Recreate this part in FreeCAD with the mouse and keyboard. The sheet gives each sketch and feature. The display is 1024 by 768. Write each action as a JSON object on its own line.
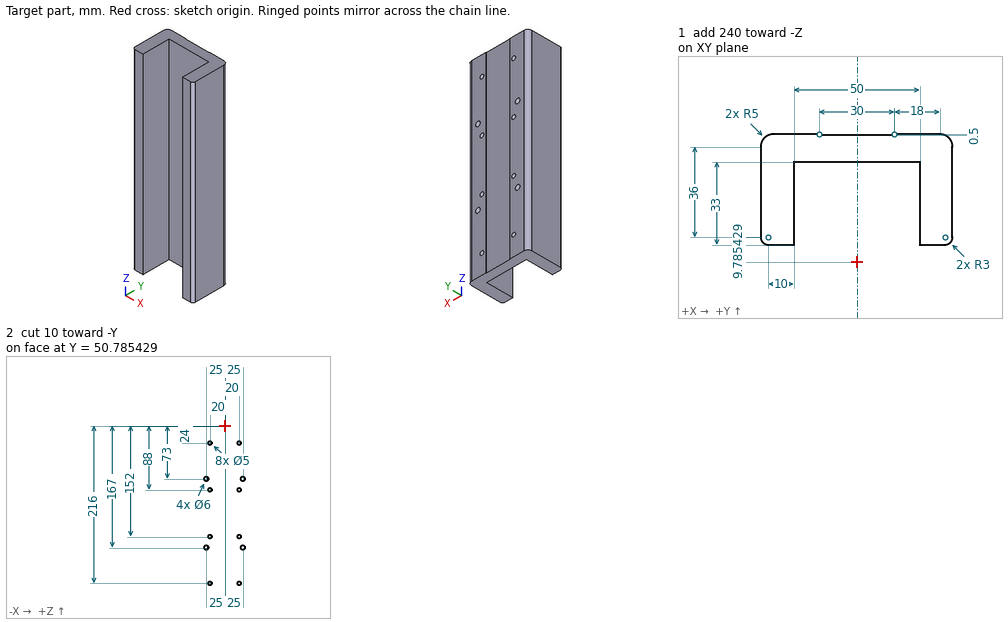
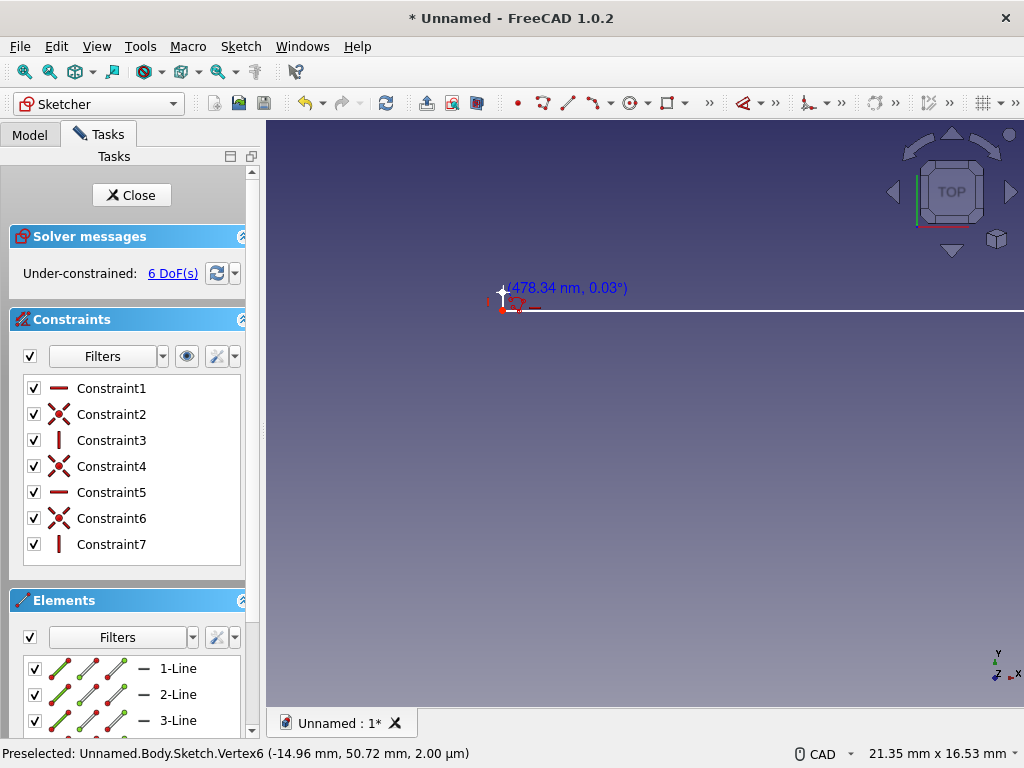
{"action": "scroll", "coordinate": [505, 291], "scroll_direction": "down", "scroll_amount": 10}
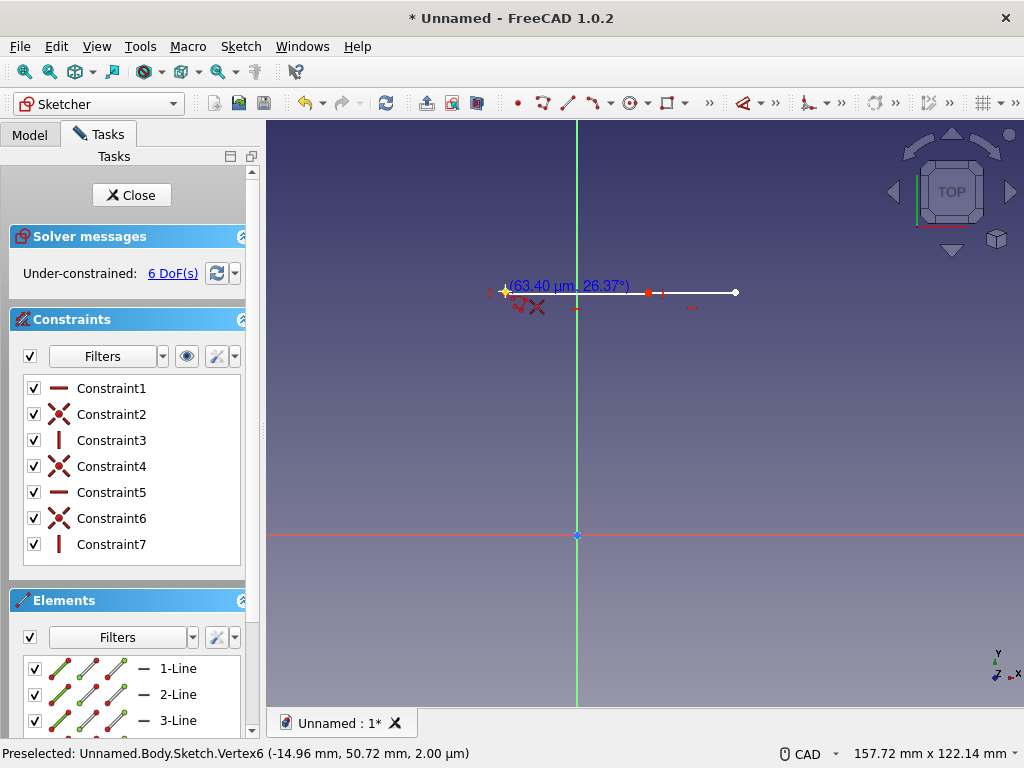
{"action": "left_click", "coordinate": [418, 291]}
{"action": "right_click", "coordinate": [418, 291]}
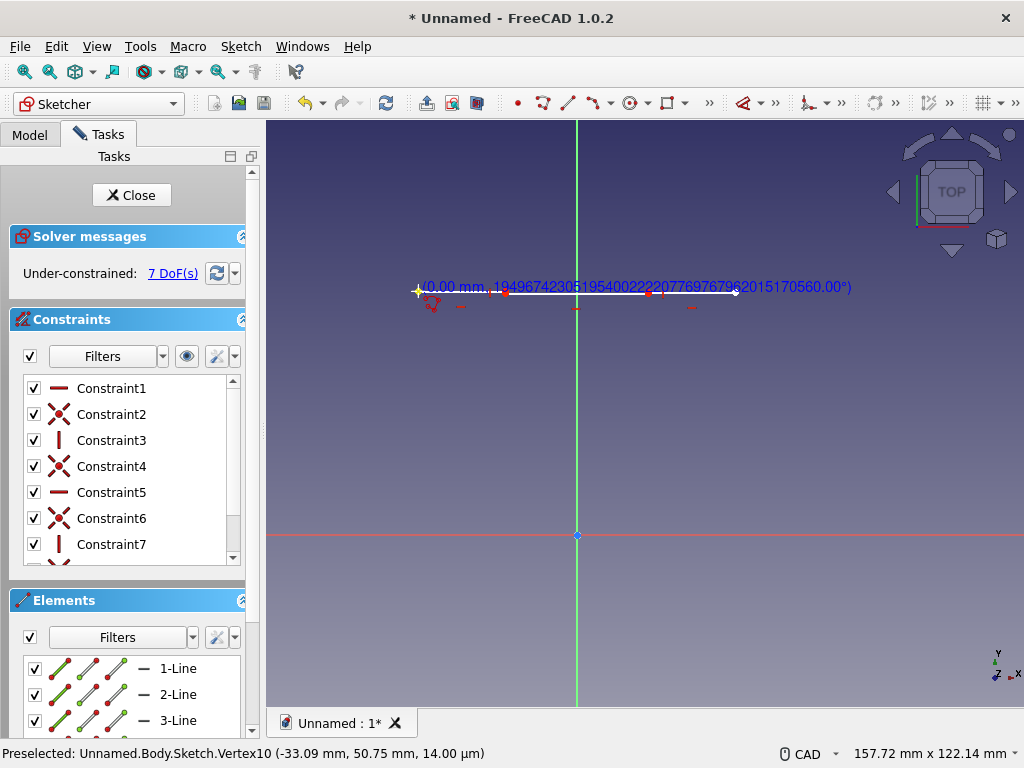
{"action": "left_click", "coordinate": [568, 104]}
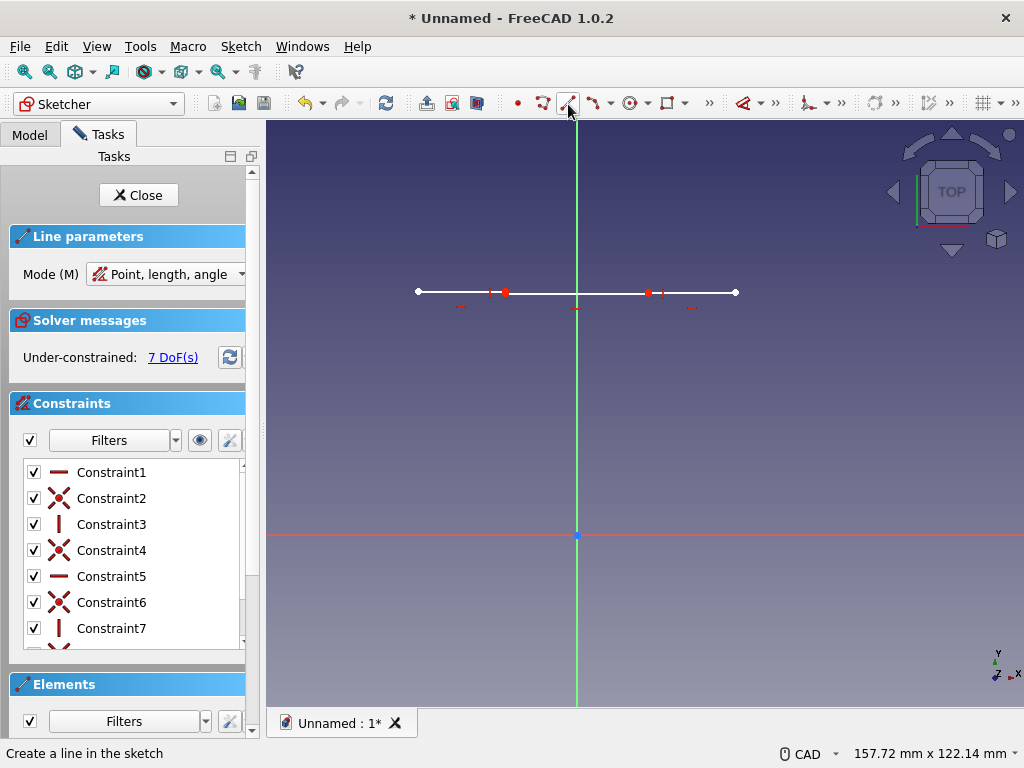
{"action": "left_click", "coordinate": [394, 315]}
{"action": "left_click", "coordinate": [394, 488]}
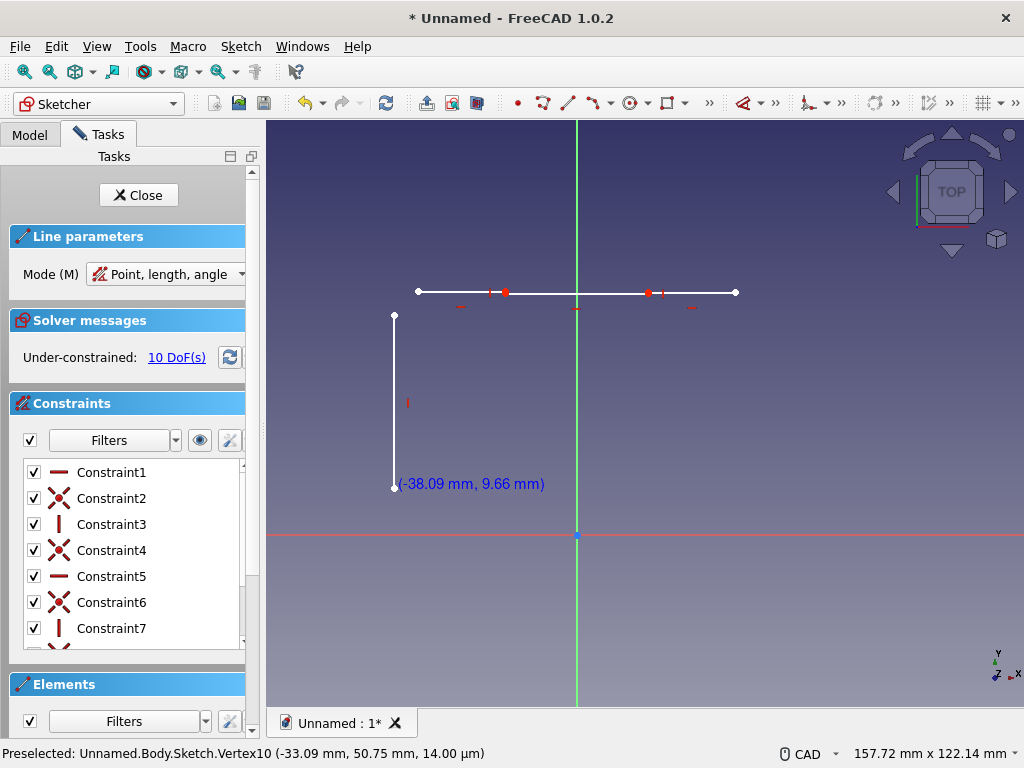
{"action": "left_click", "coordinate": [543, 104]}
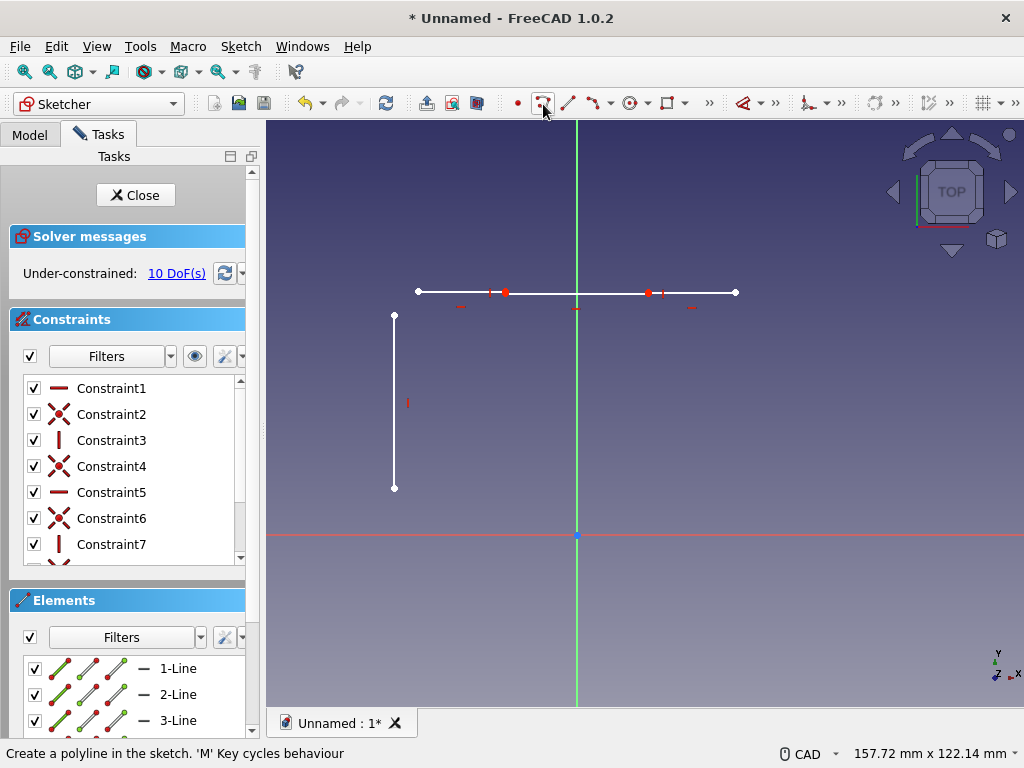
{"action": "left_click", "coordinate": [409, 503]}
{"action": "left_click", "coordinate": [457, 503]}
{"action": "left_click", "coordinate": [457, 344]}
{"action": "left_click", "coordinate": [697, 344]}
{"action": "left_click", "coordinate": [697, 503]}
{"action": "left_click", "coordinate": [745, 503]}
{"action": "right_click", "coordinate": [745, 503]}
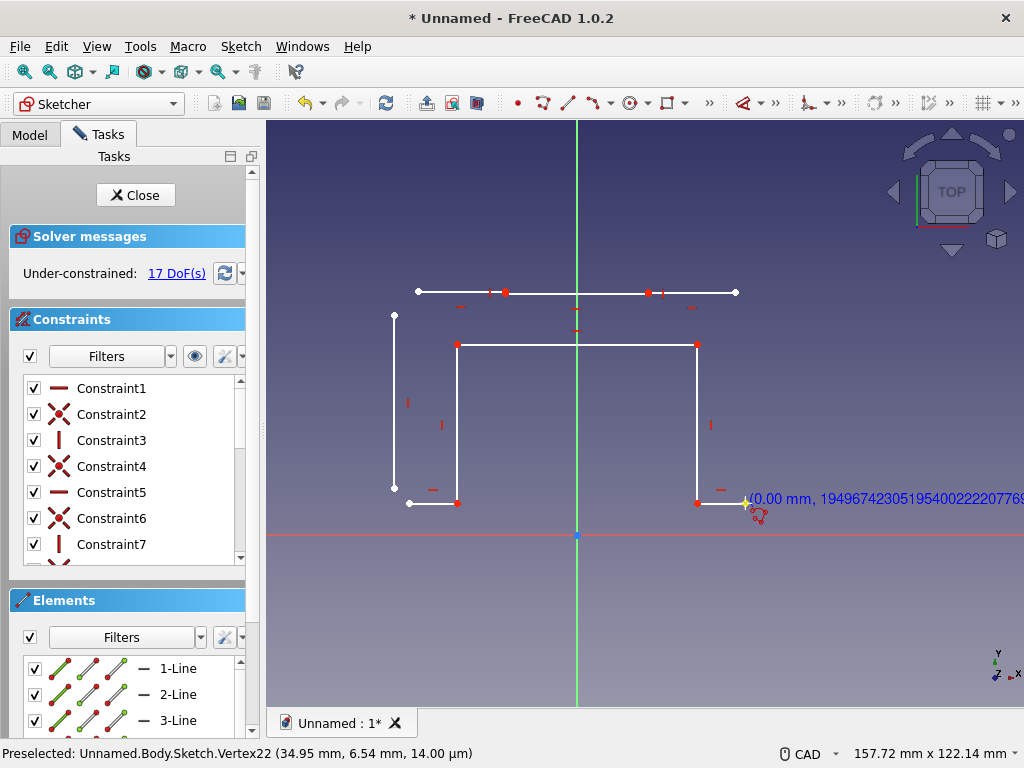
{"action": "left_click", "coordinate": [568, 104]}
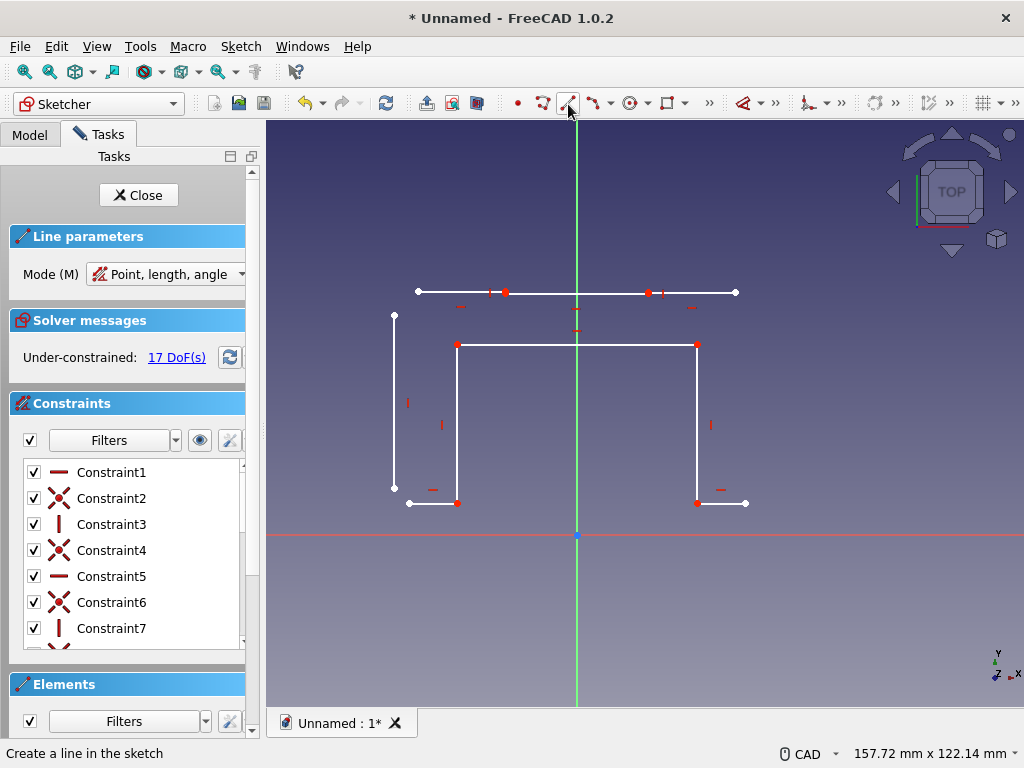
{"action": "left_click", "coordinate": [760, 488]}
{"action": "left_click", "coordinate": [760, 315]}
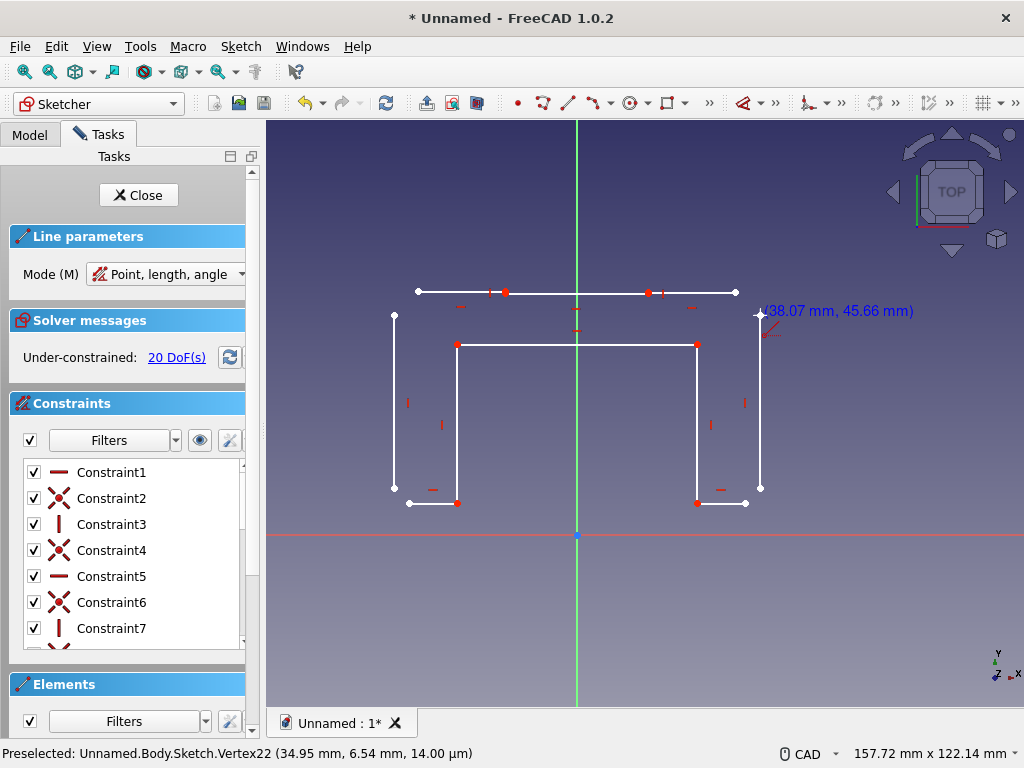
{"action": "left_click", "coordinate": [592, 104]}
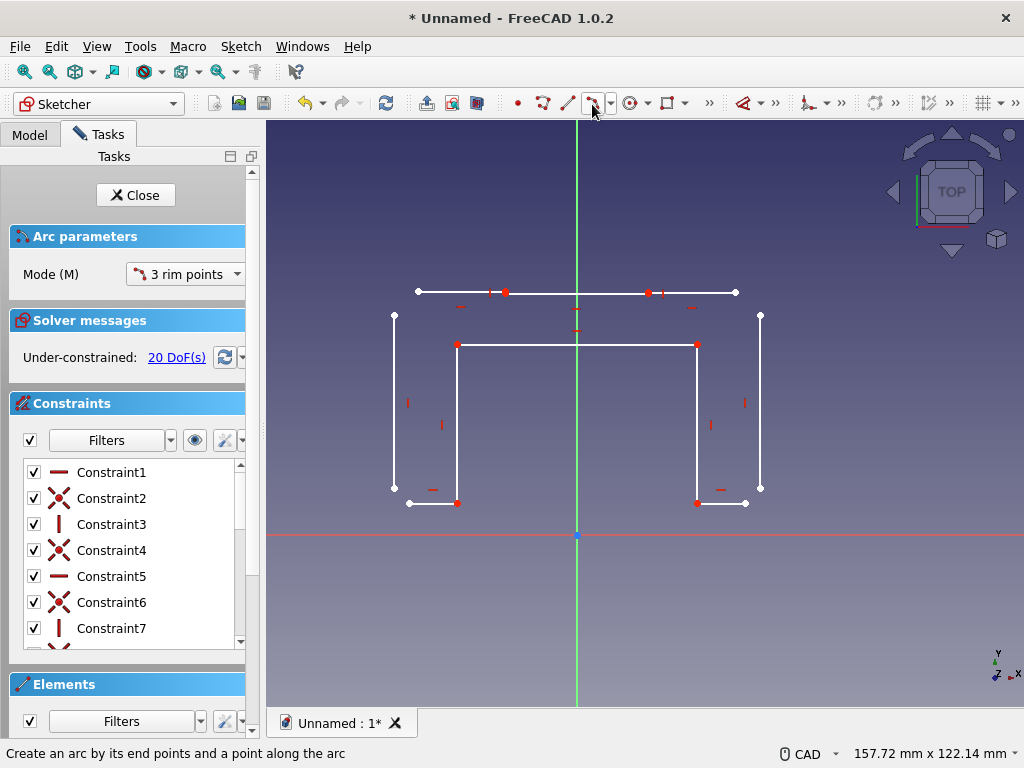
{"action": "left_click", "coordinate": [418, 292]}
{"action": "left_click", "coordinate": [394, 316]}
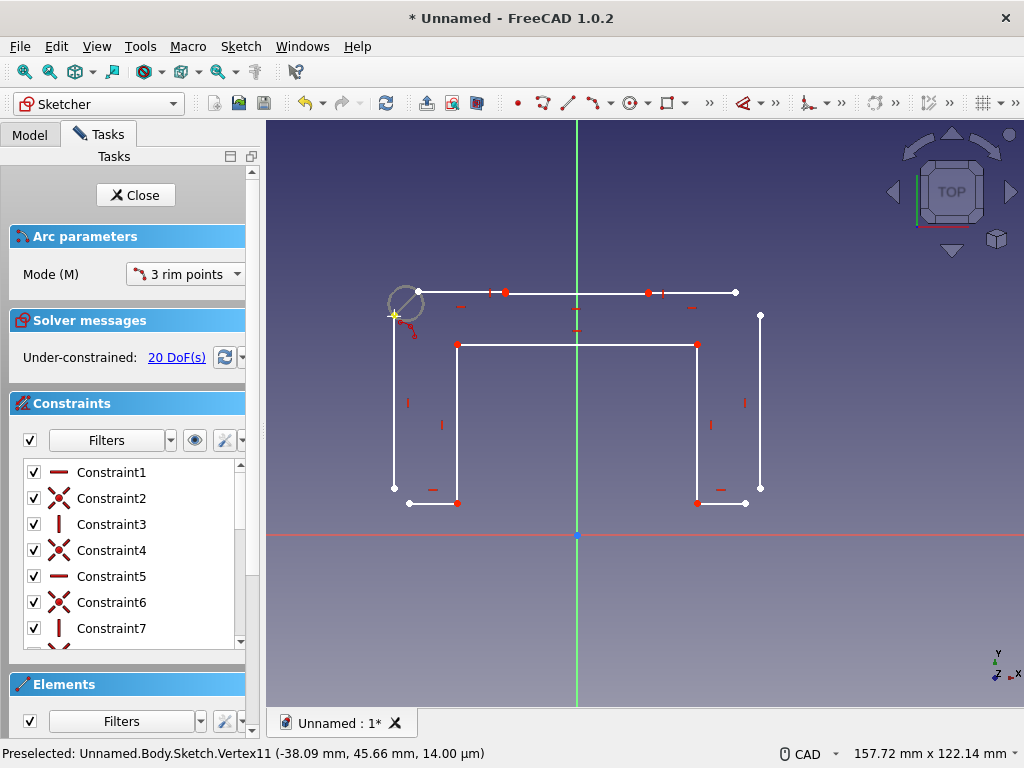
{"action": "scroll", "coordinate": [401, 298], "scroll_direction": "up", "scroll_amount": 5}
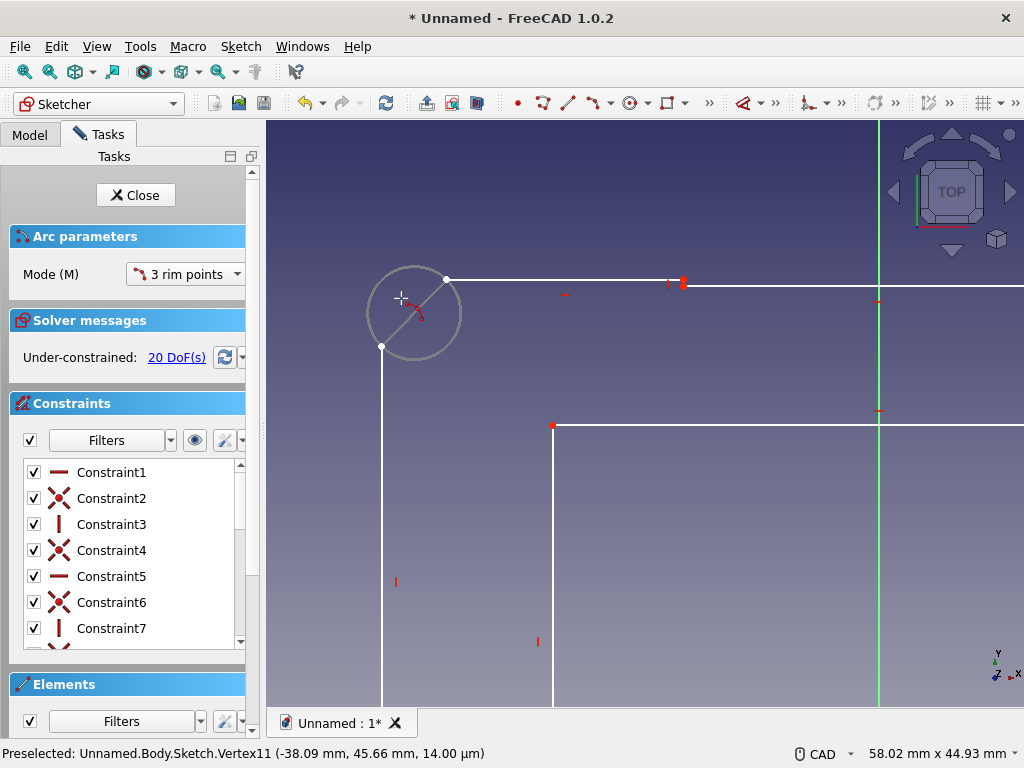
{"action": "left_click", "coordinate": [402, 299]}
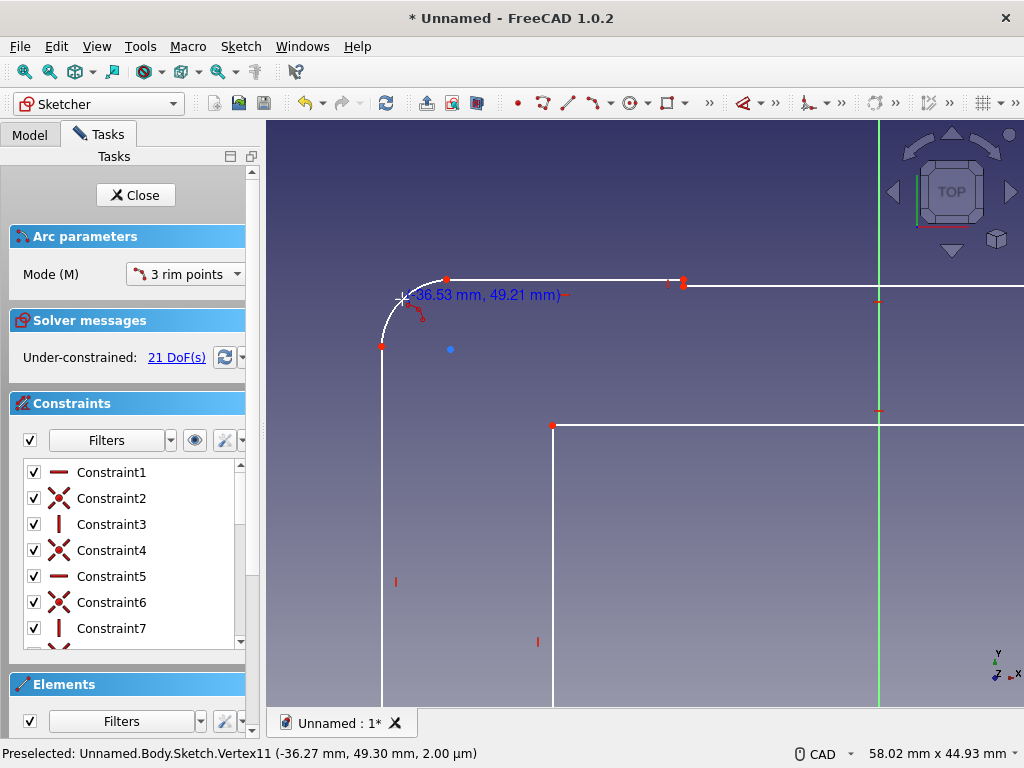
{"action": "scroll", "coordinate": [400, 298], "scroll_direction": "down", "scroll_amount": 5}